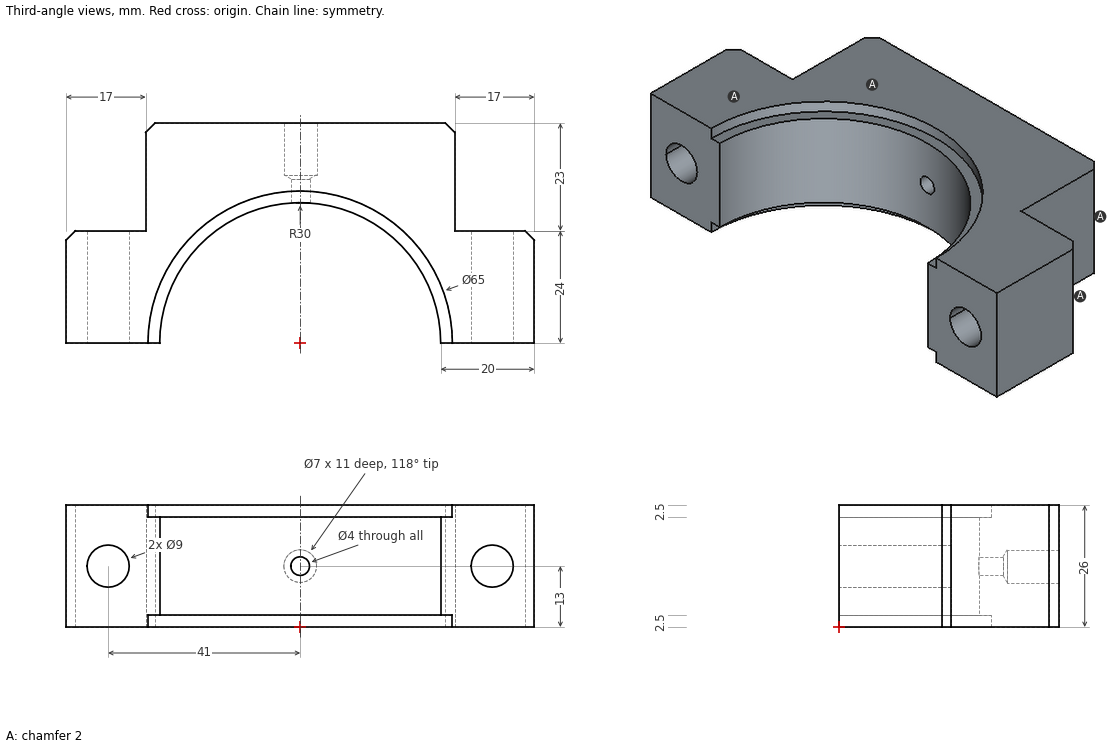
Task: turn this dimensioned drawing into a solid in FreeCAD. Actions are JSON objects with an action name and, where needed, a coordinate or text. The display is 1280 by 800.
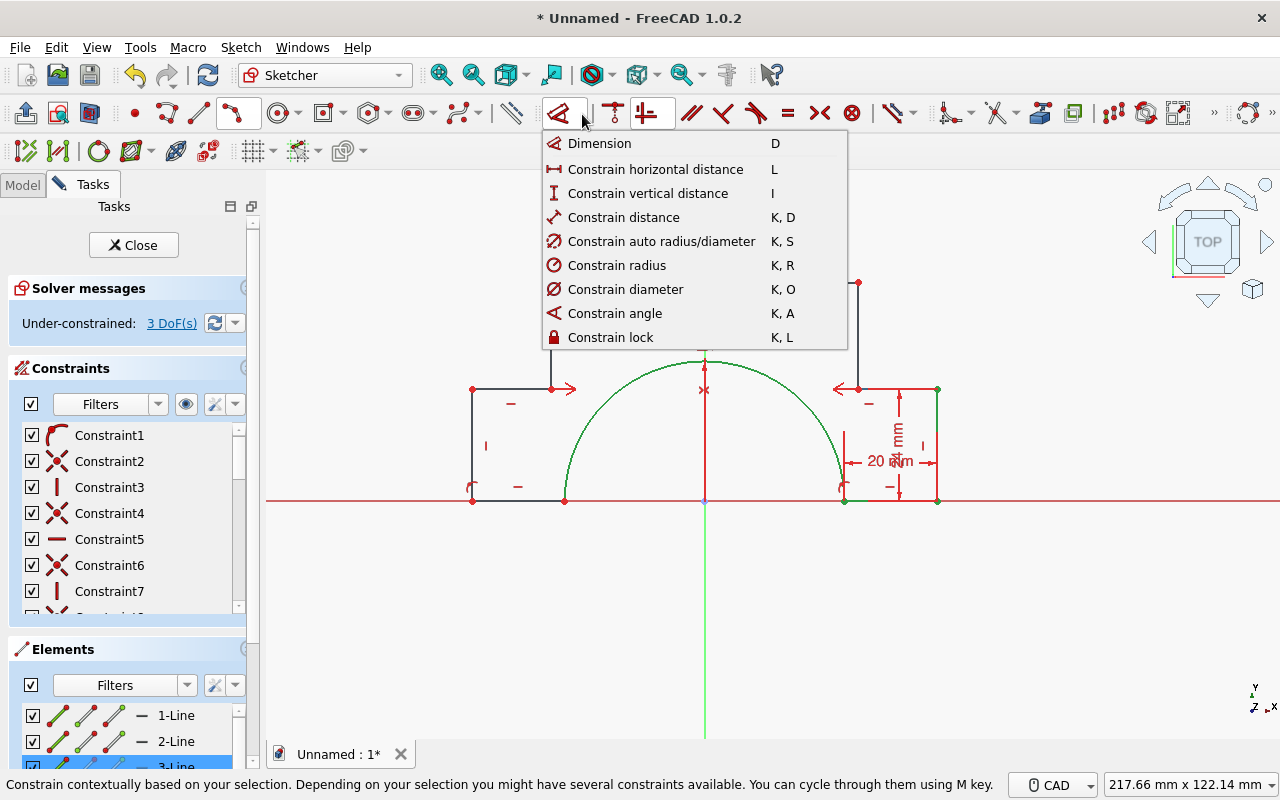
{"action": "left_click", "coordinate": [695, 169]}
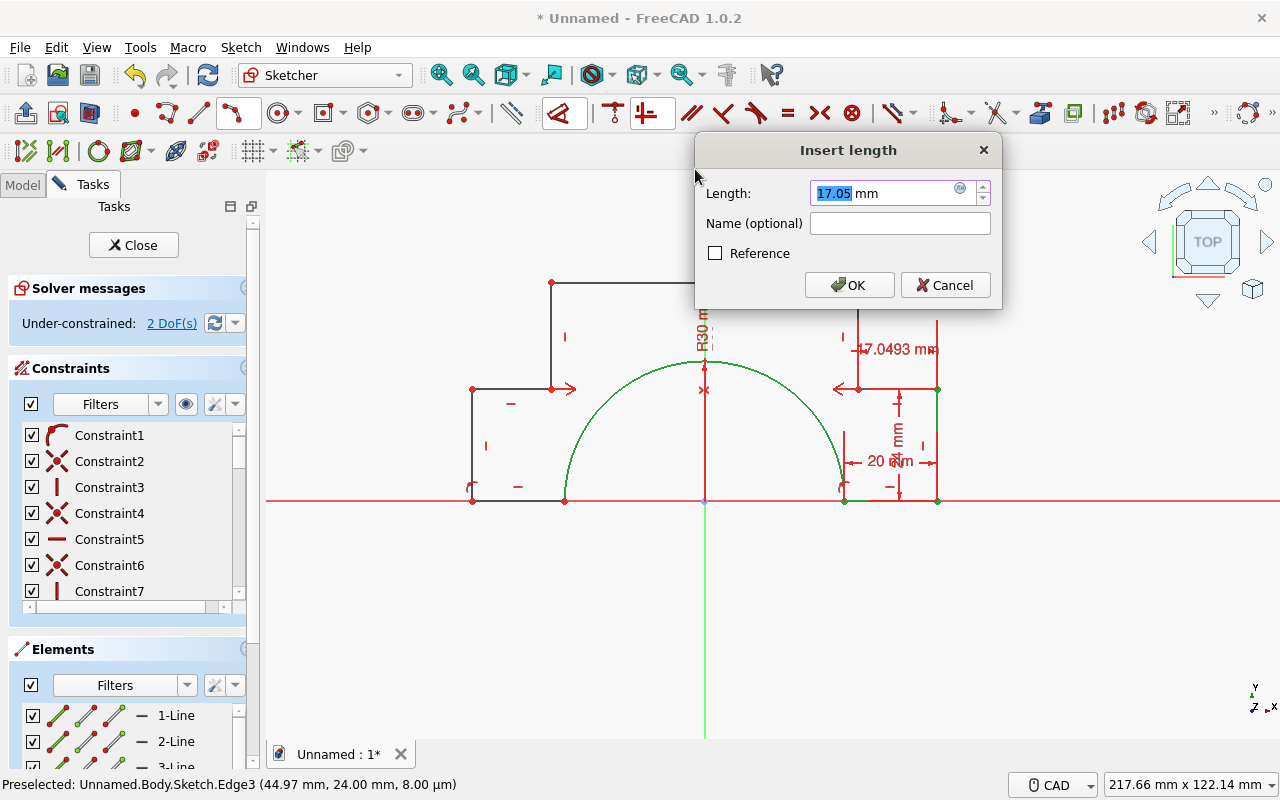
{"action": "type", "text": "17"}
{"action": "key", "text": "Return"}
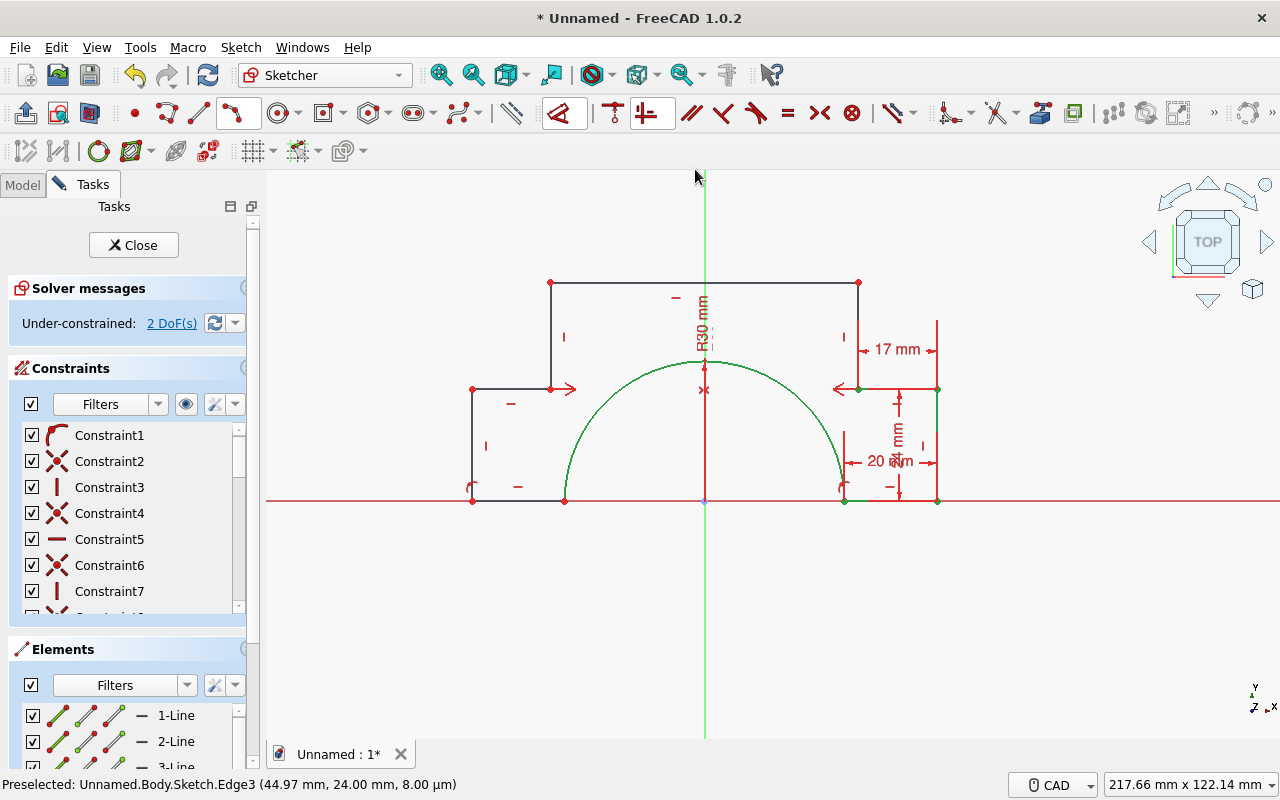
{"action": "left_click", "coordinate": [858, 357]}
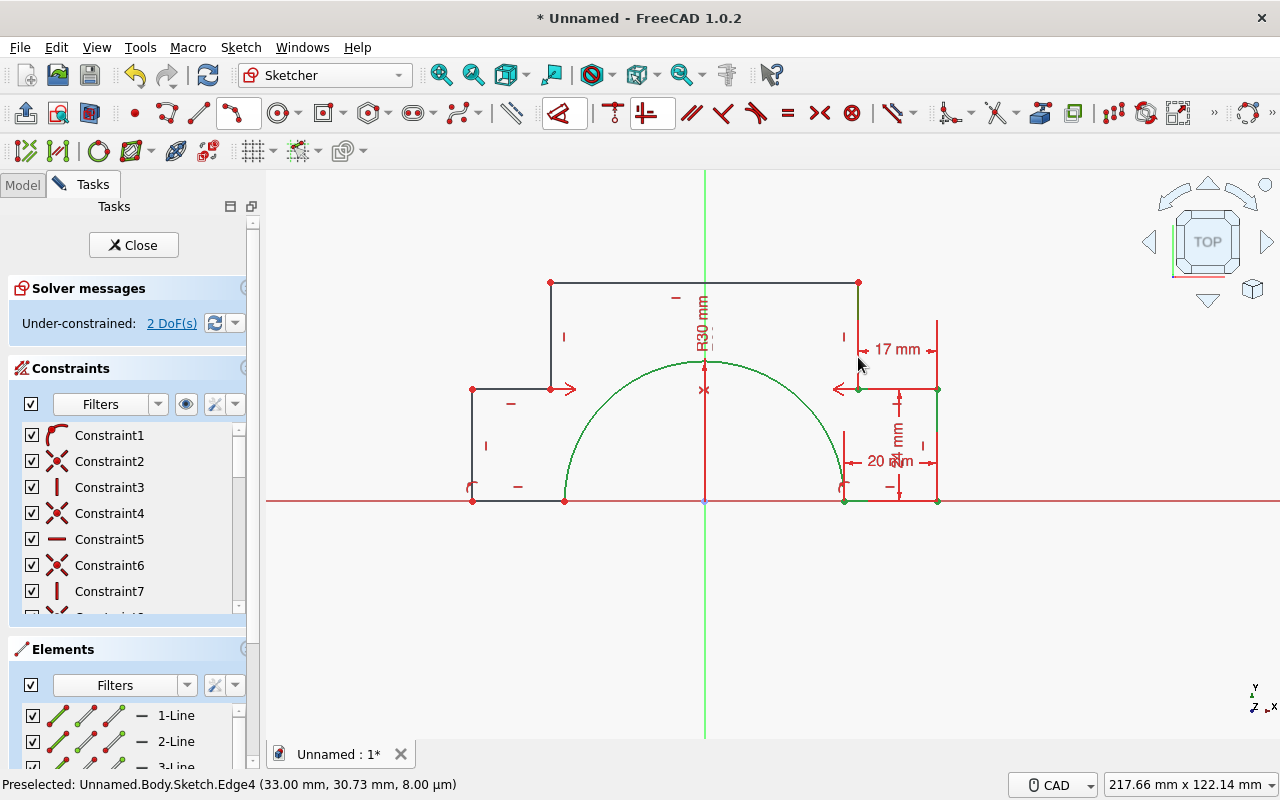
{"action": "key", "text": "i"}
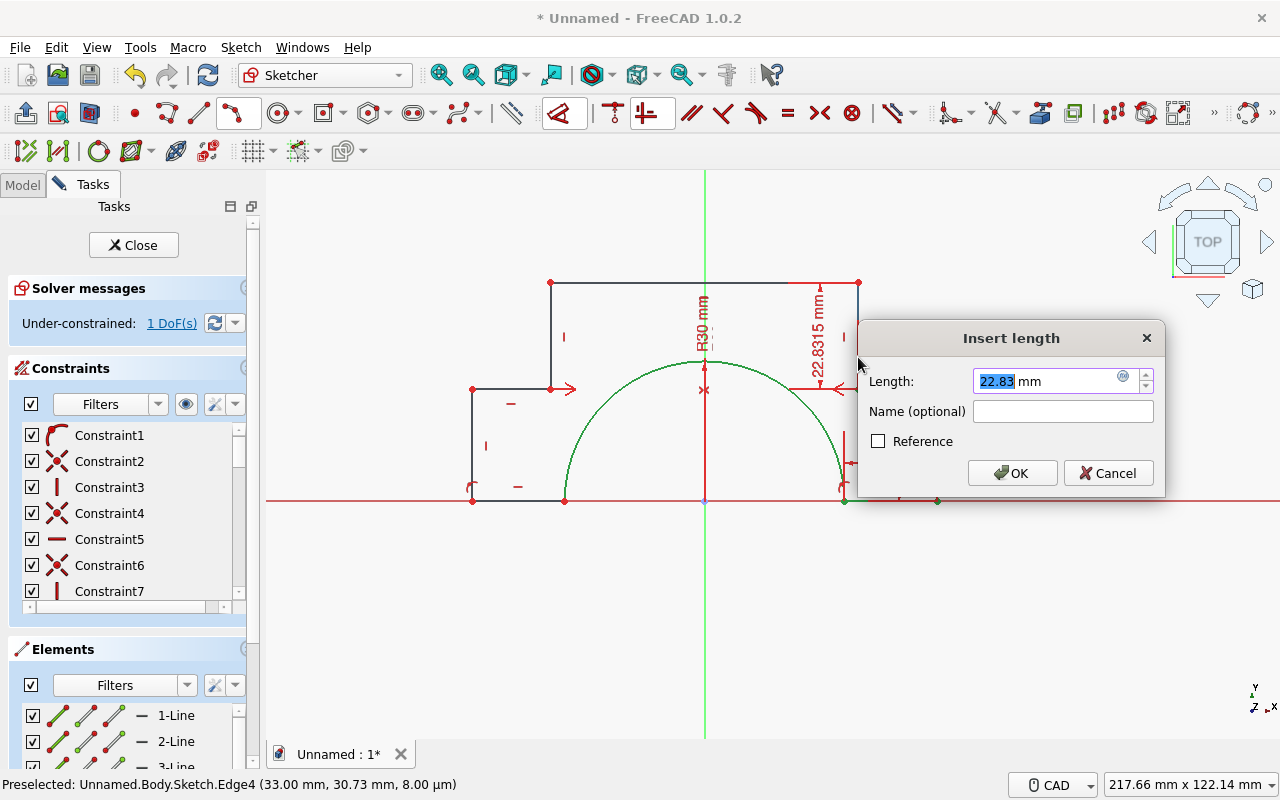
{"action": "type", "text": "23"}
{"action": "key", "text": "Return"}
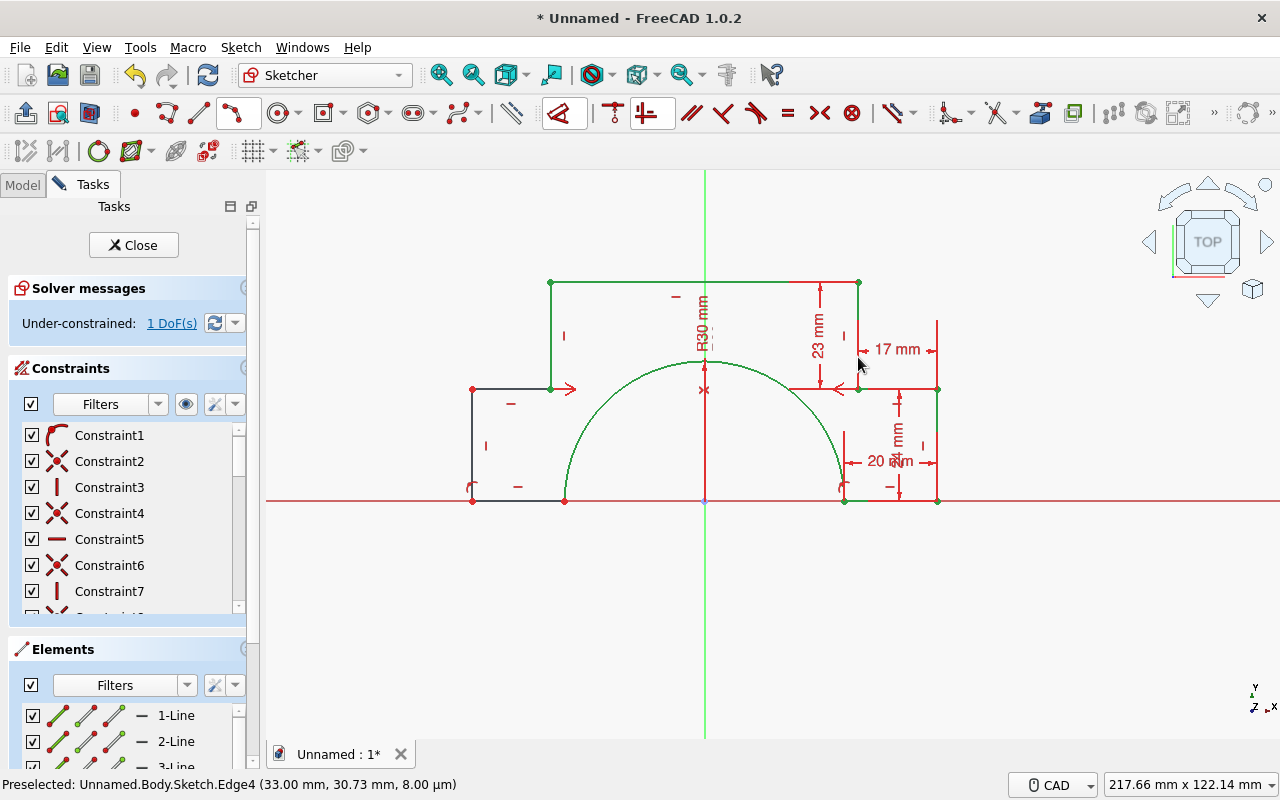
{"action": "left_click", "coordinate": [527, 389]}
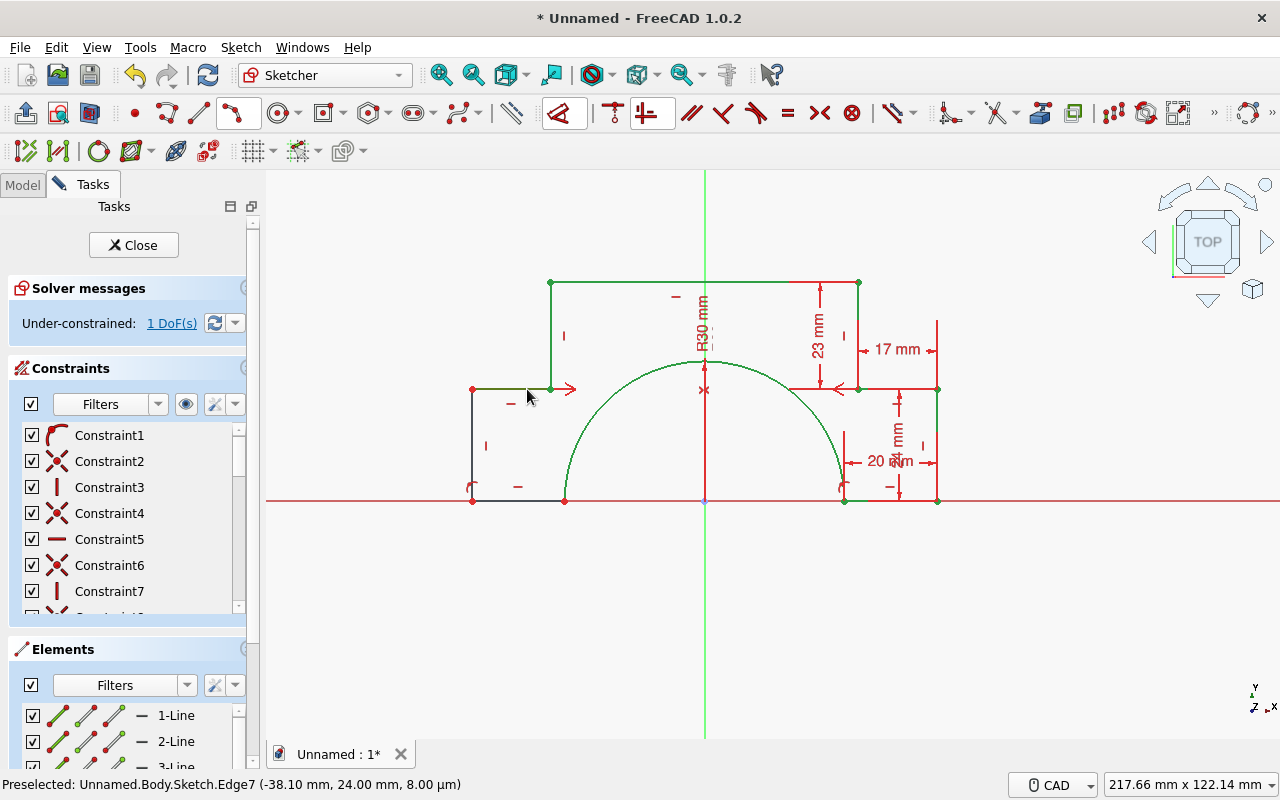
{"action": "key", "text": "l"}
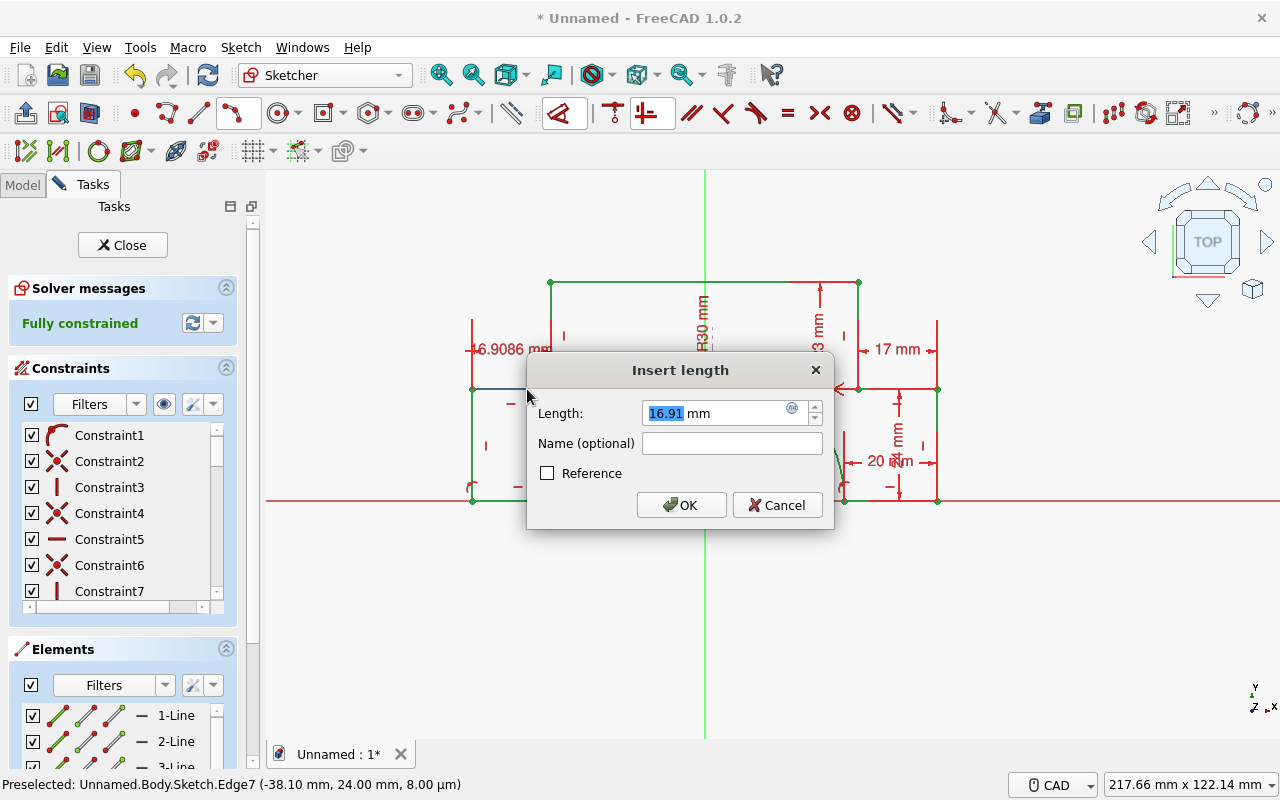
{"action": "type", "text": "17"}
{"action": "key", "text": "Return"}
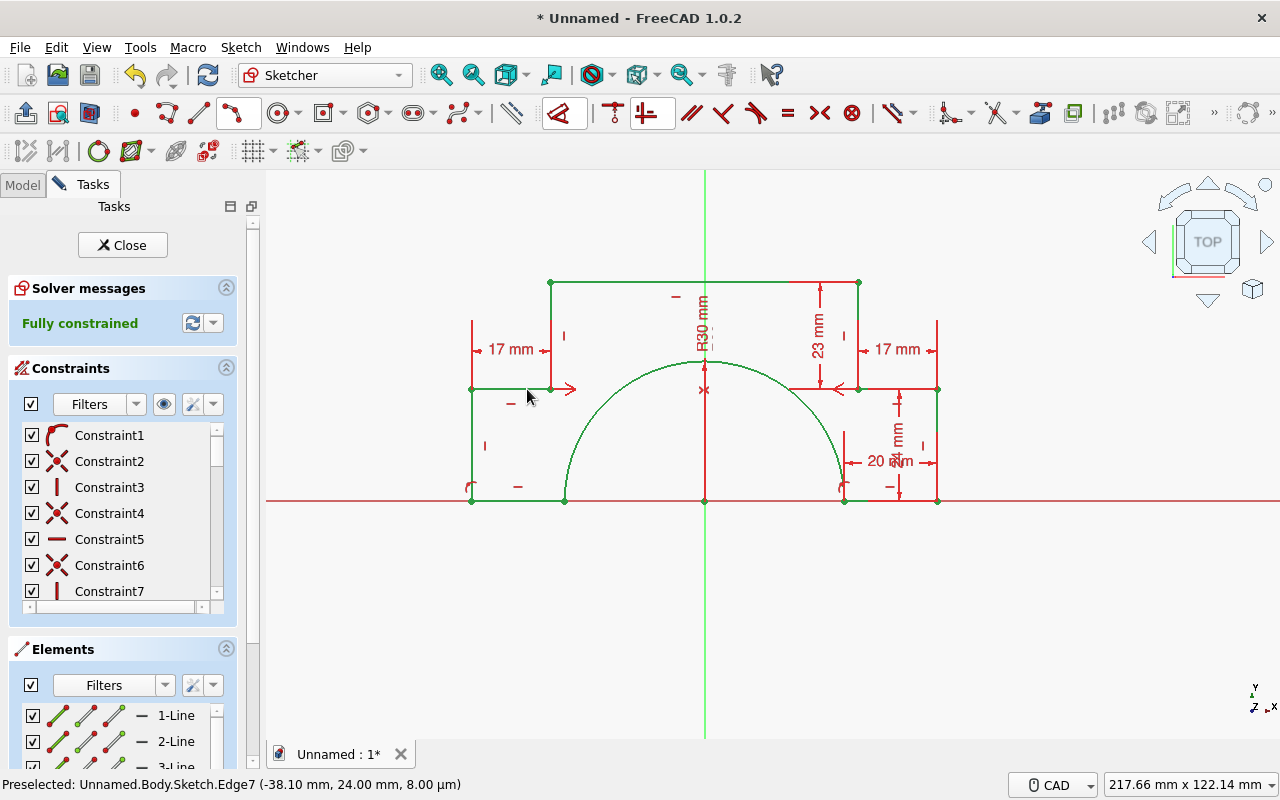
{"action": "left_click", "coordinate": [123, 245]}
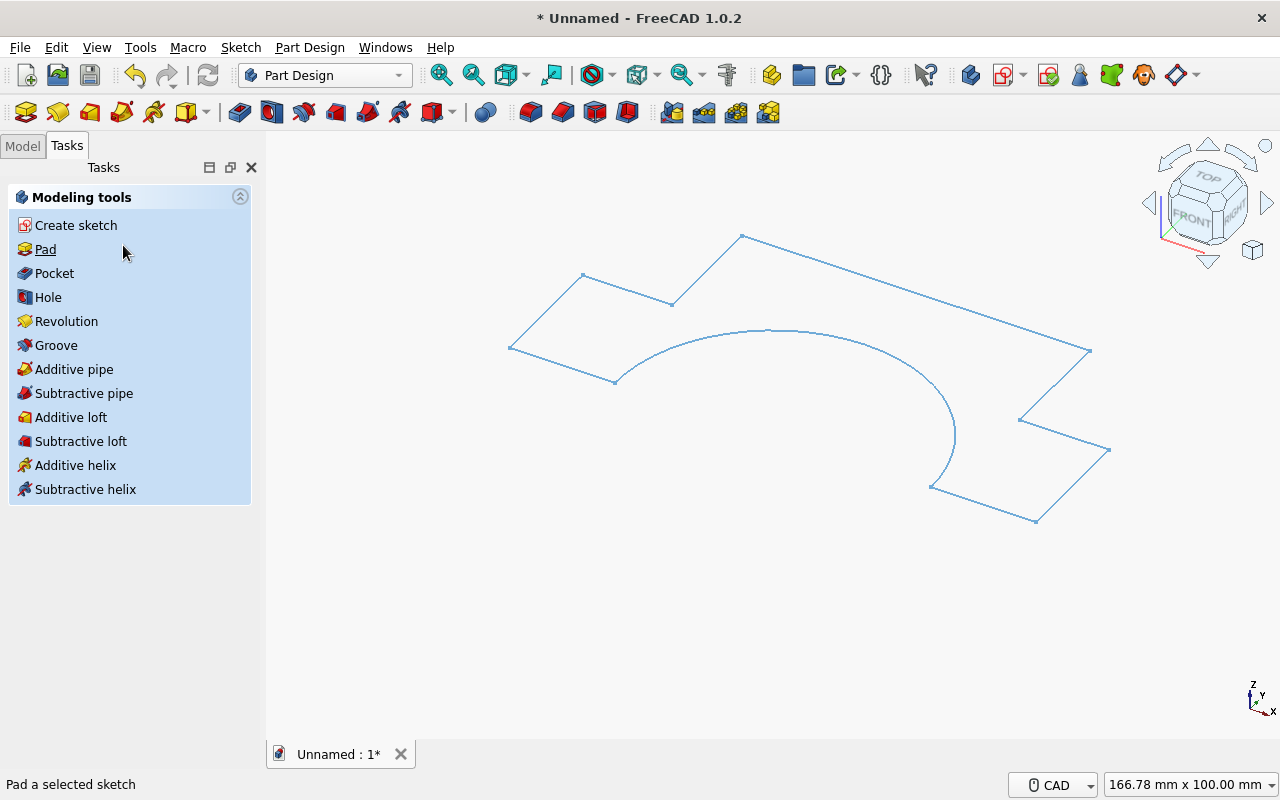
{"action": "left_click", "coordinate": [26, 112]}